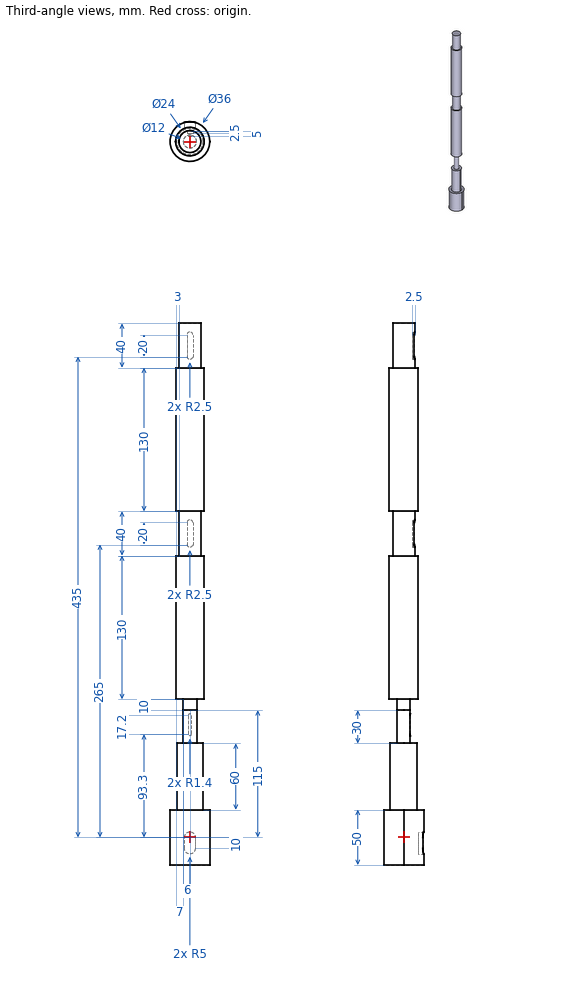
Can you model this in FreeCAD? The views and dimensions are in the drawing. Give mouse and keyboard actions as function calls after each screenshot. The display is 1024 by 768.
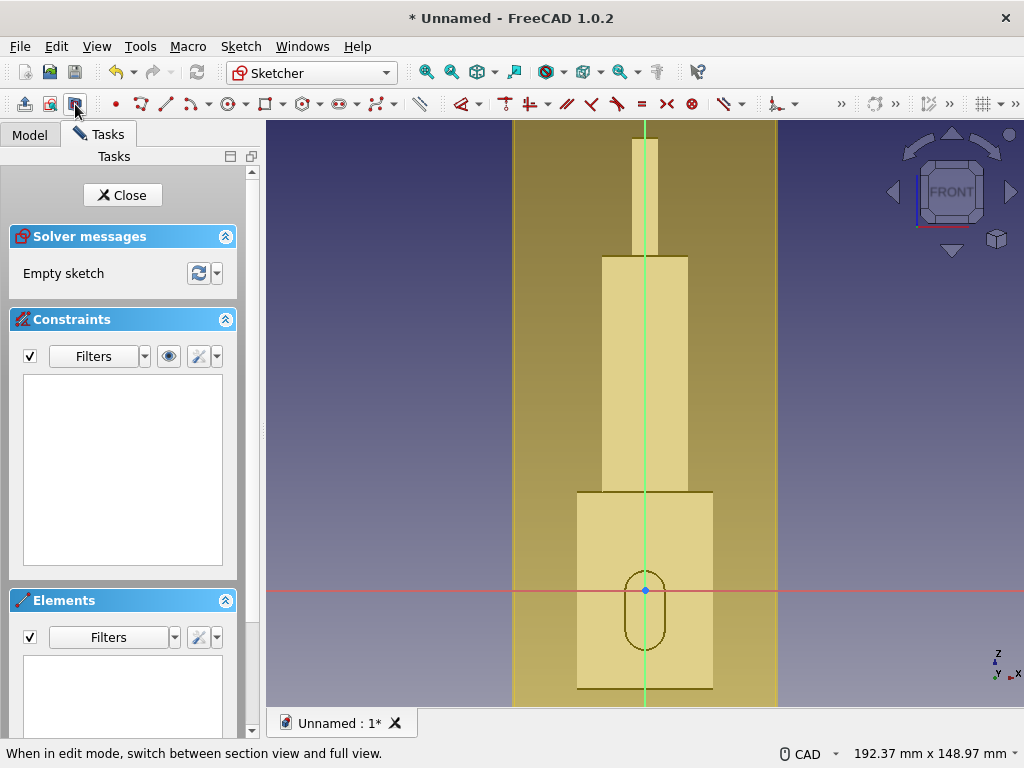
scroll(576, 414, down, 5)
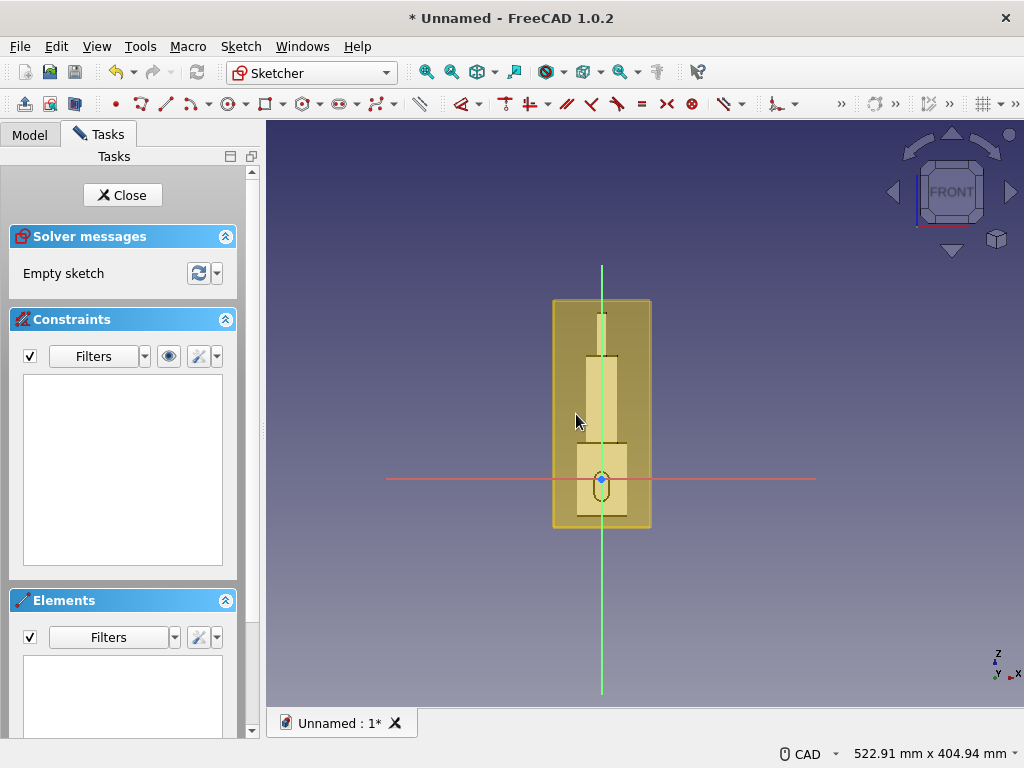
scroll(604, 325, up, 13)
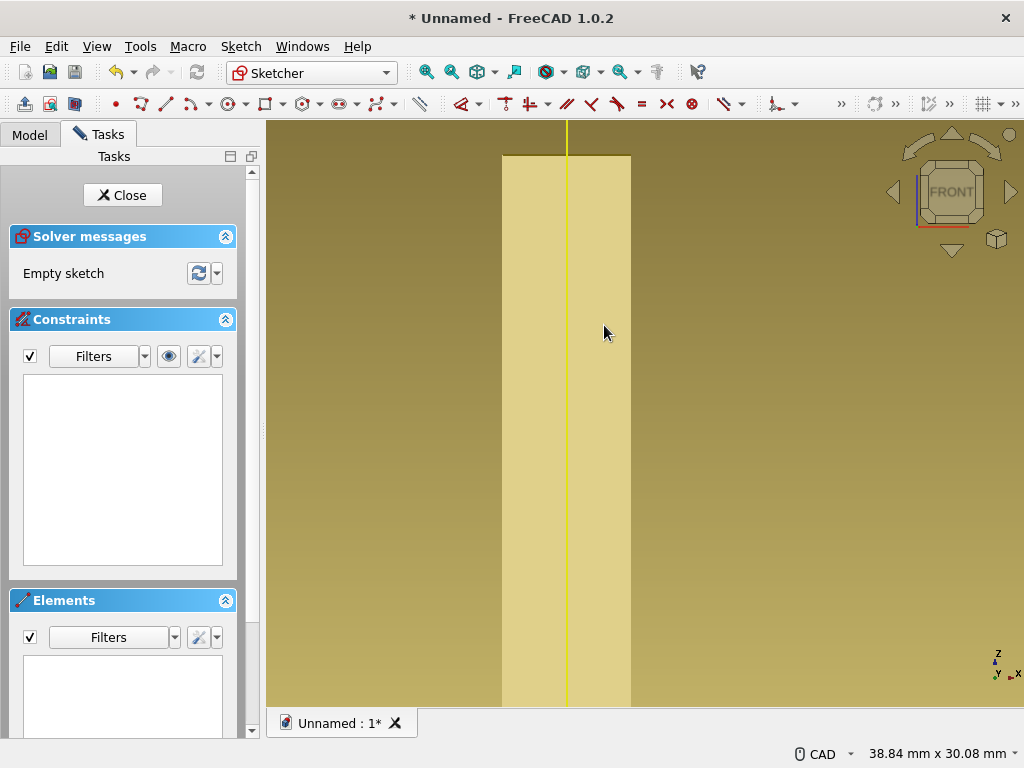
click(338, 104)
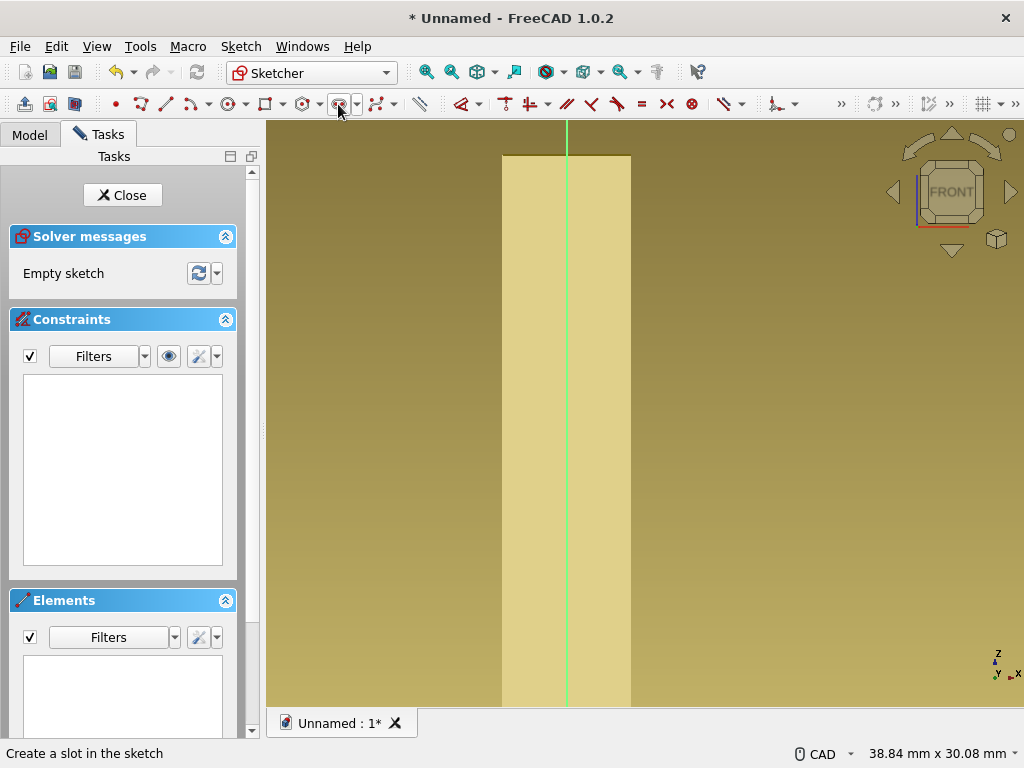
click(567, 578)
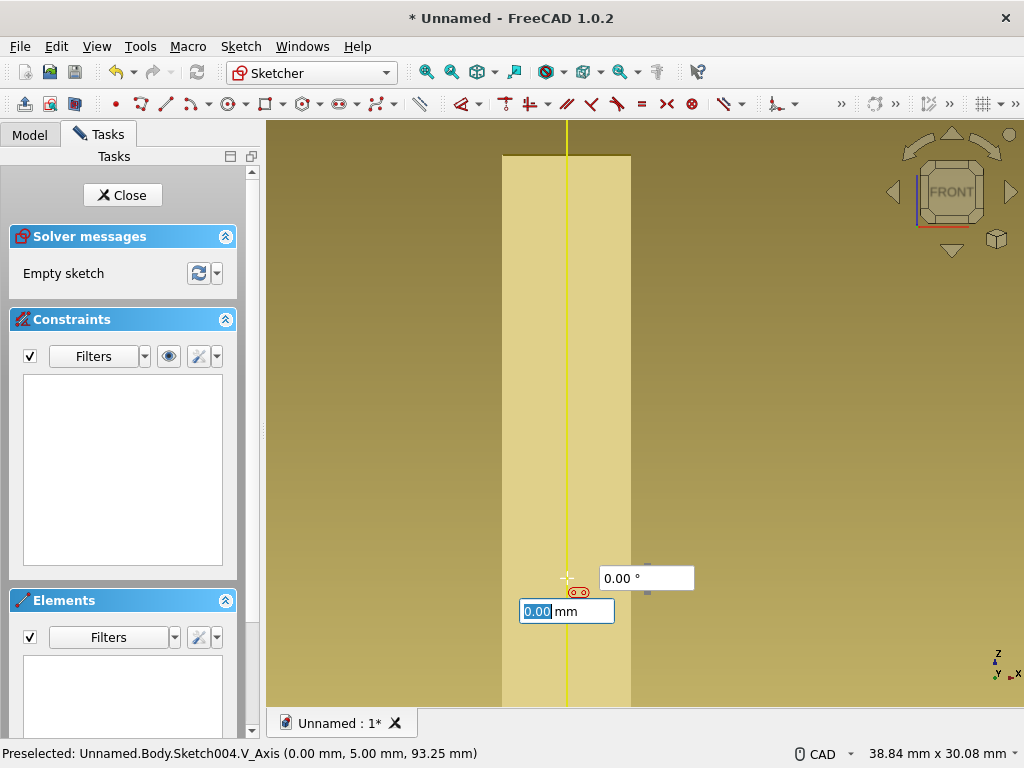
click(576, 242)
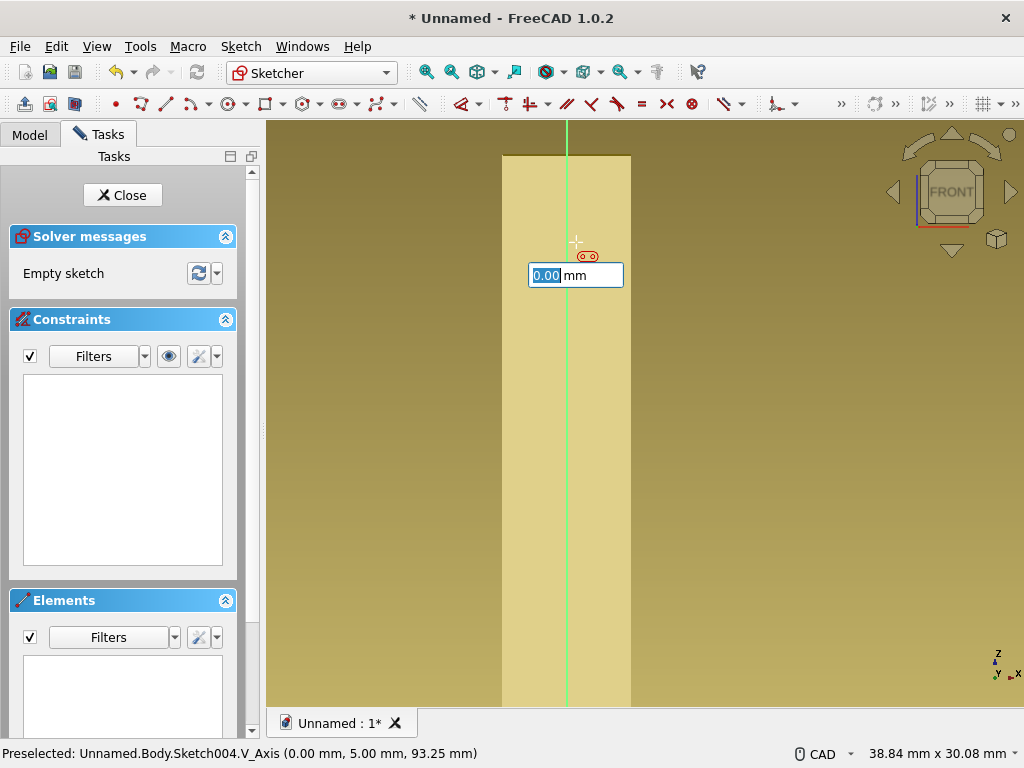
click(594, 410)
key(Escape)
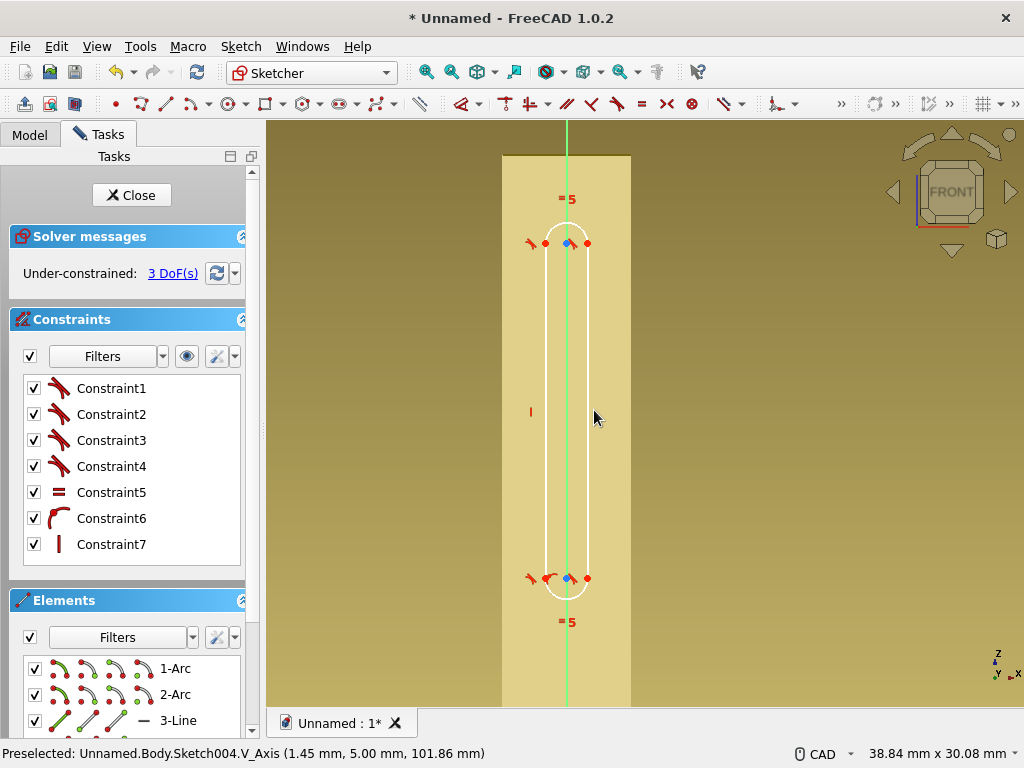
click(460, 104)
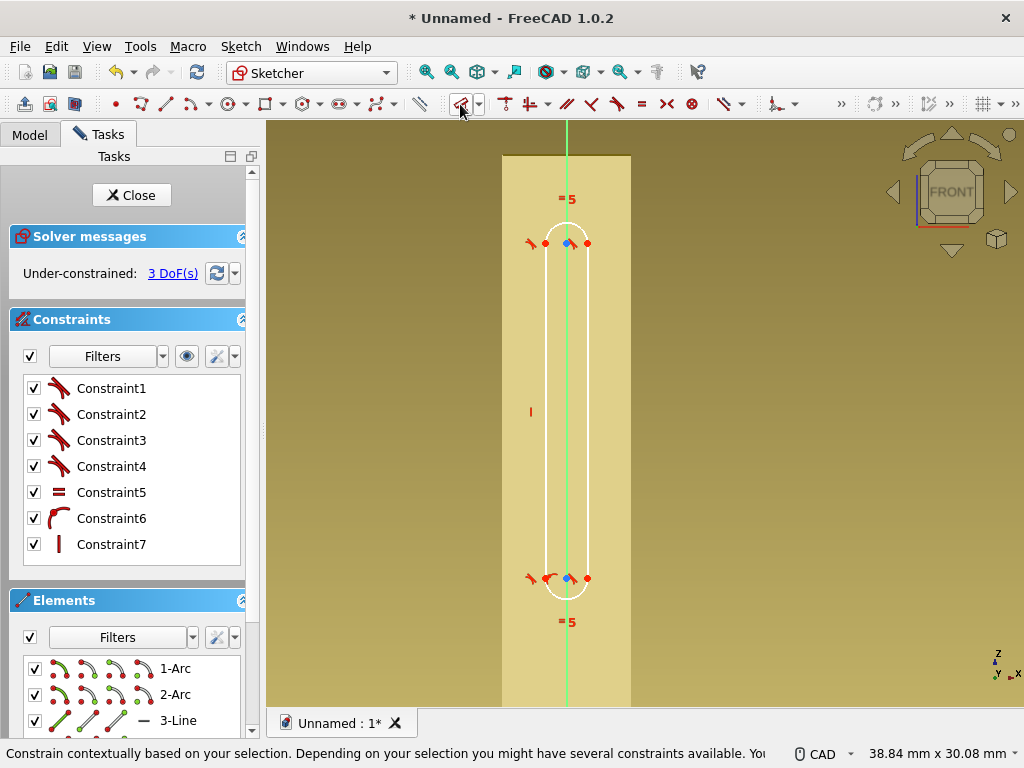
scroll(554, 595, up, 2)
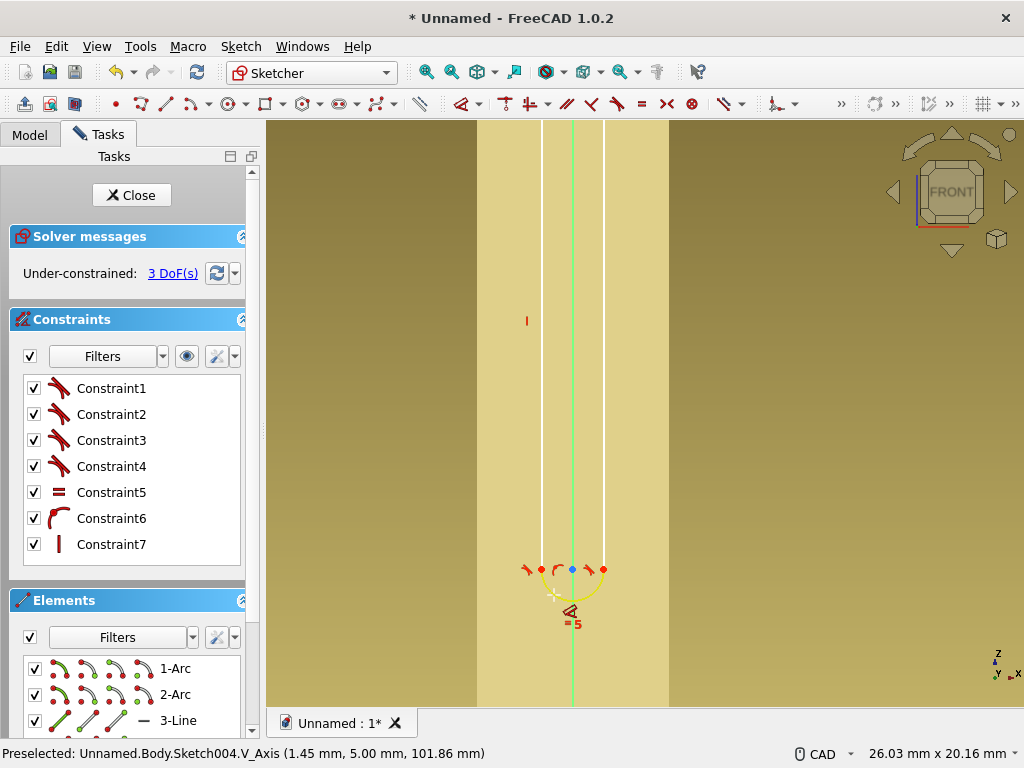
click(554, 595)
click(535, 621)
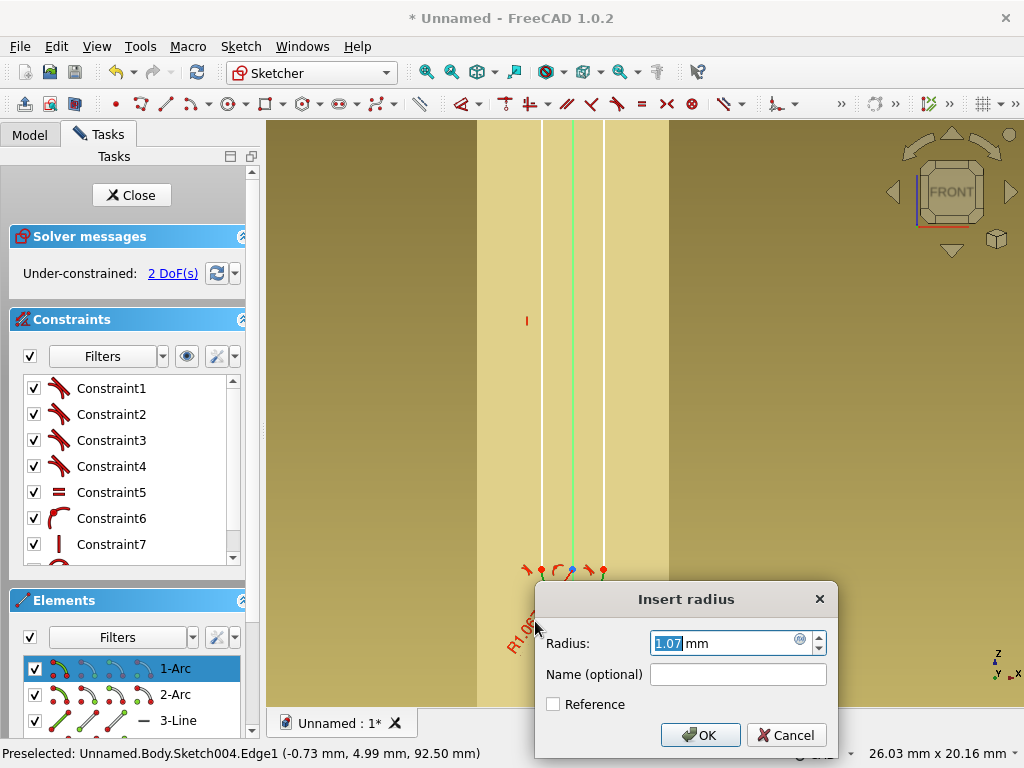
text(1.4)
key(Return)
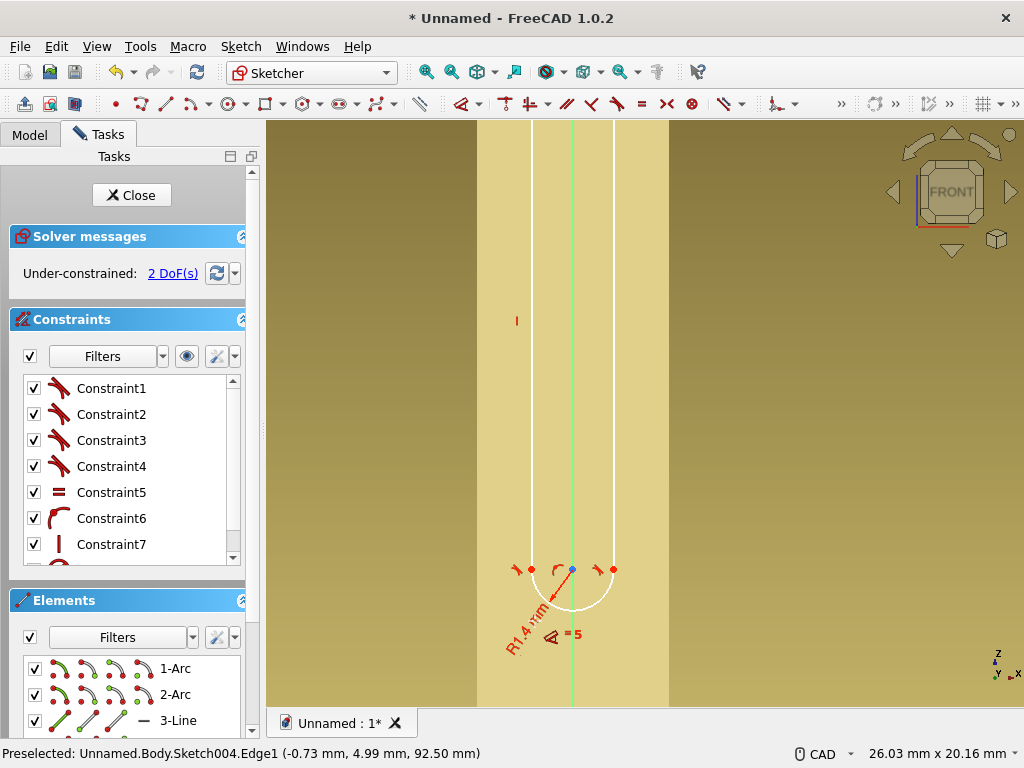
click(532, 420)
click(498, 359)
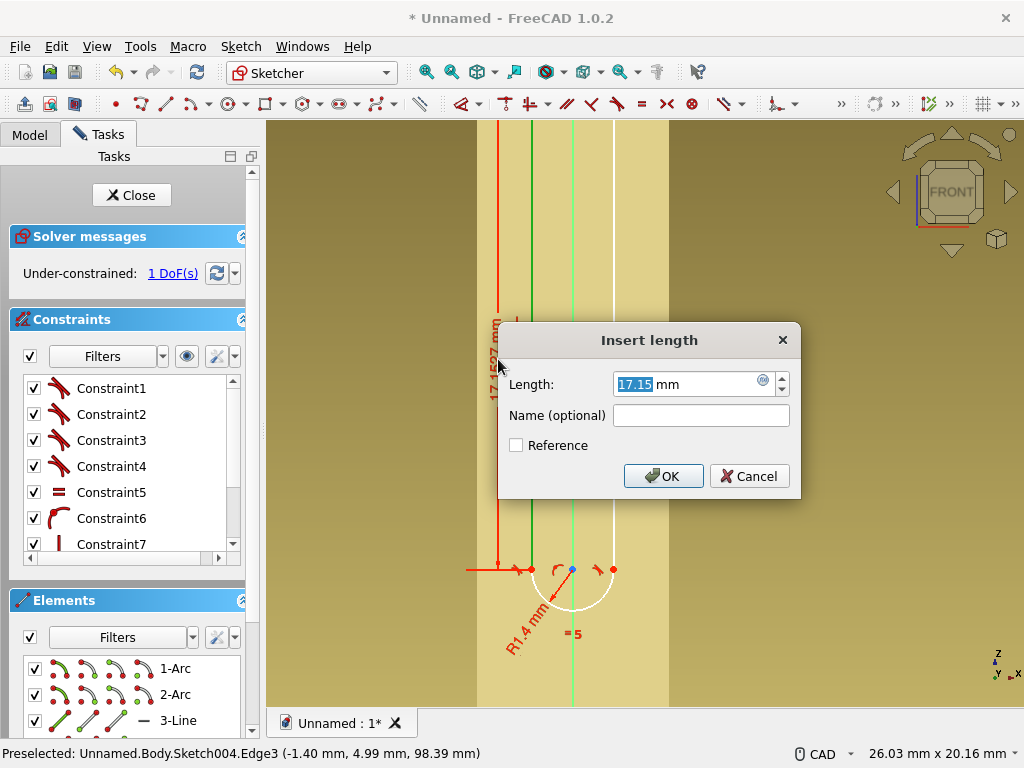
text(17.2)
key(Return)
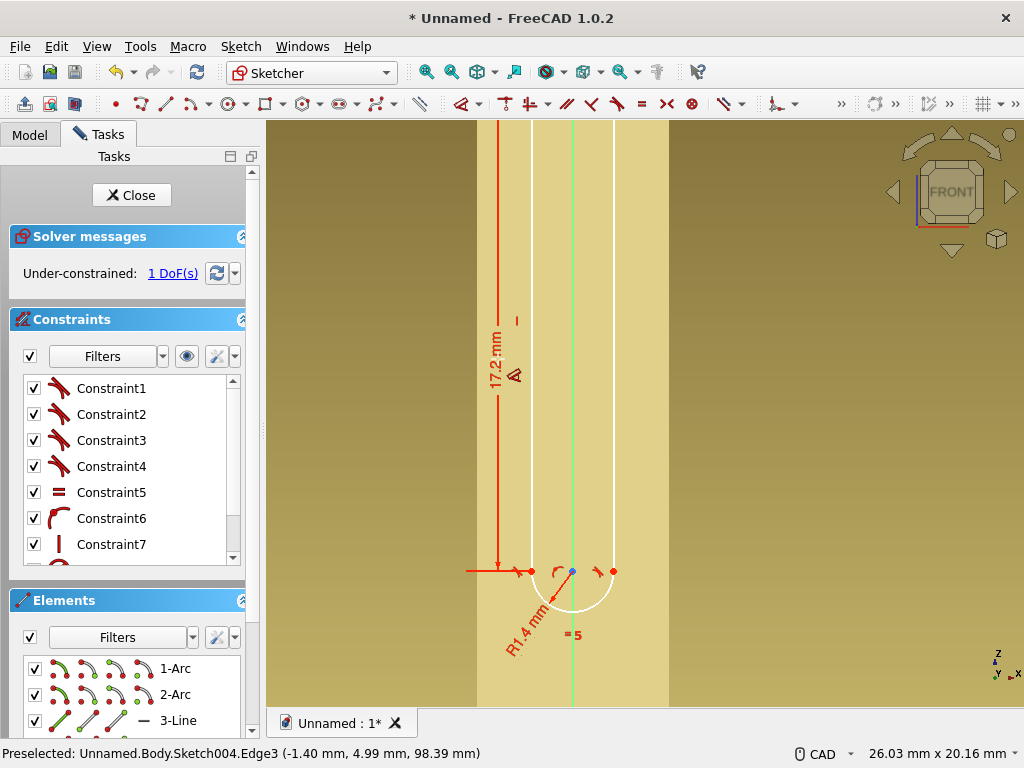
click(532, 571)
click(498, 600)